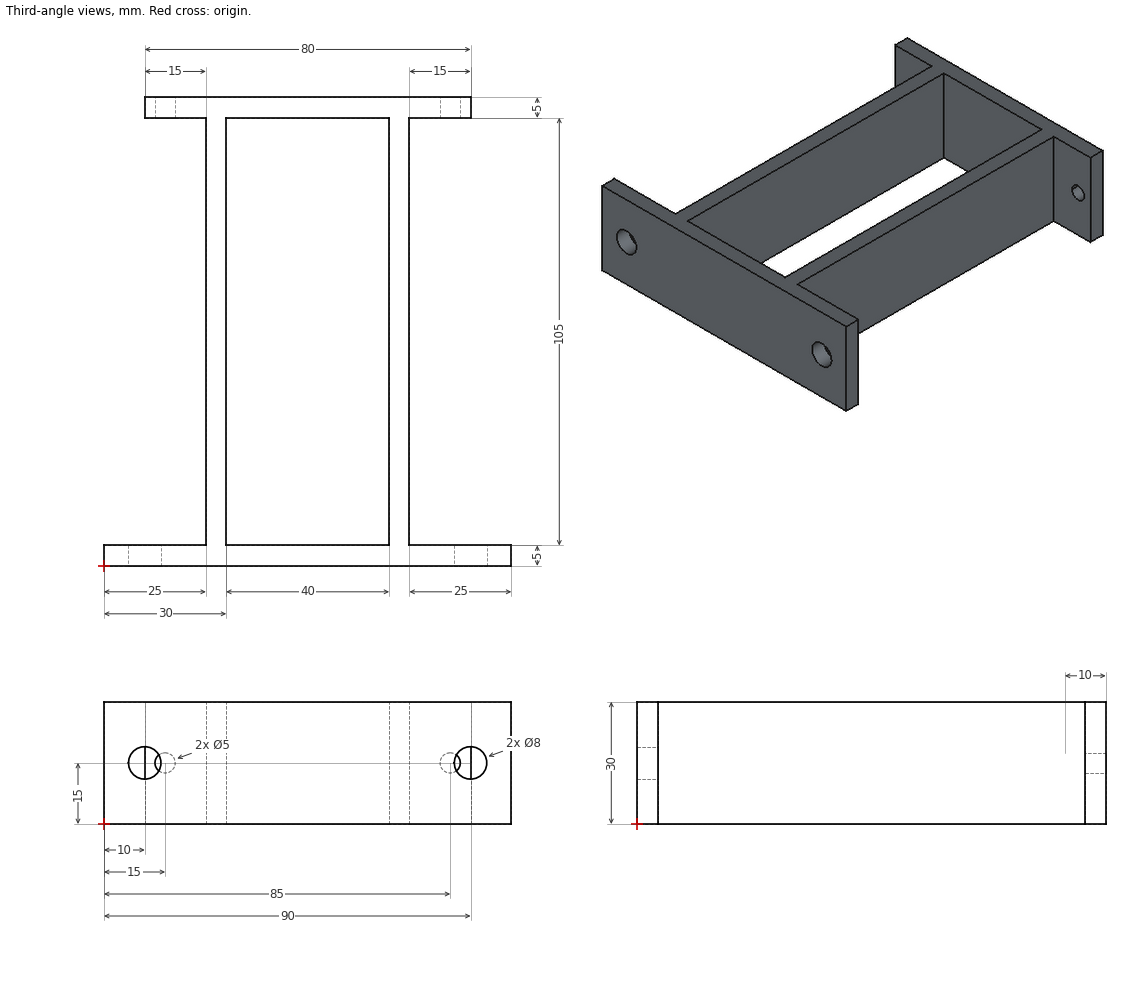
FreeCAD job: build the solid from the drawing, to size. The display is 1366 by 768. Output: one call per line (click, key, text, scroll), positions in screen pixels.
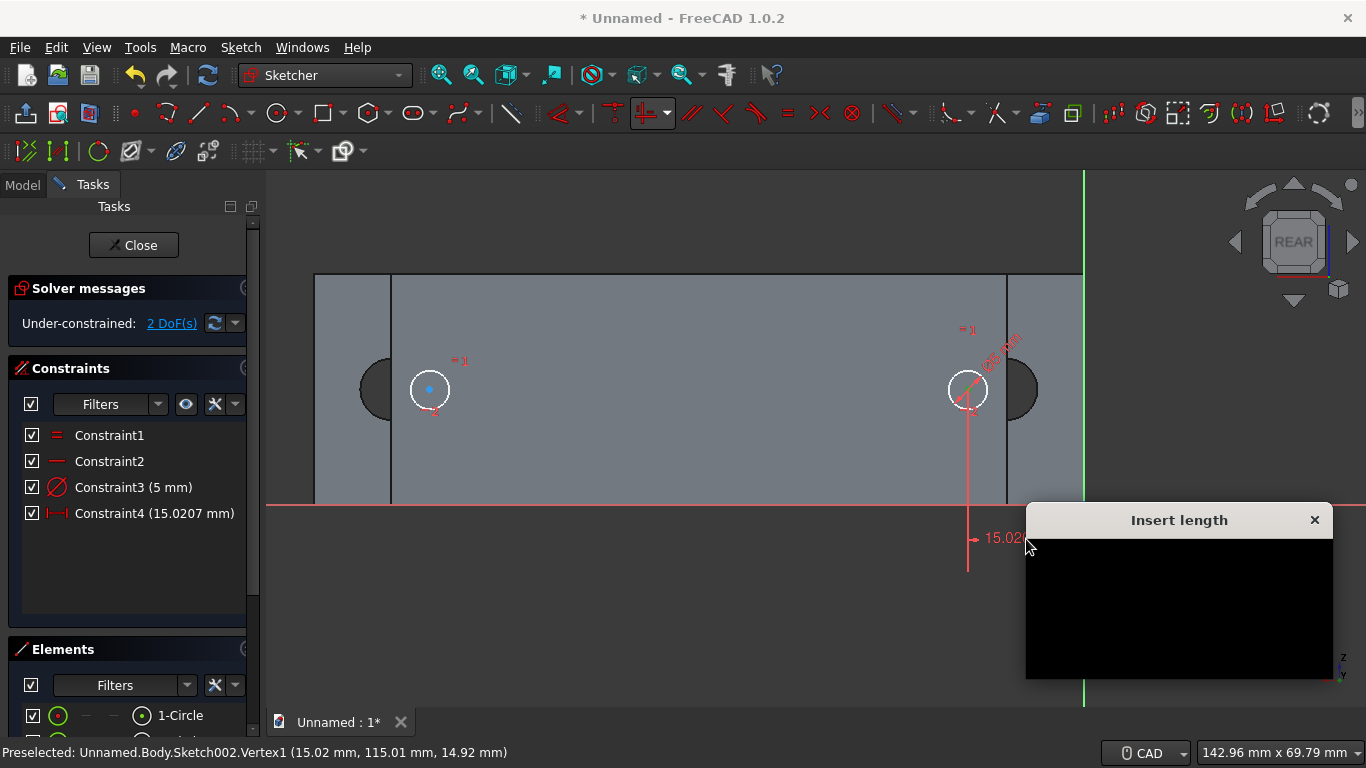
text(15)
key(Return)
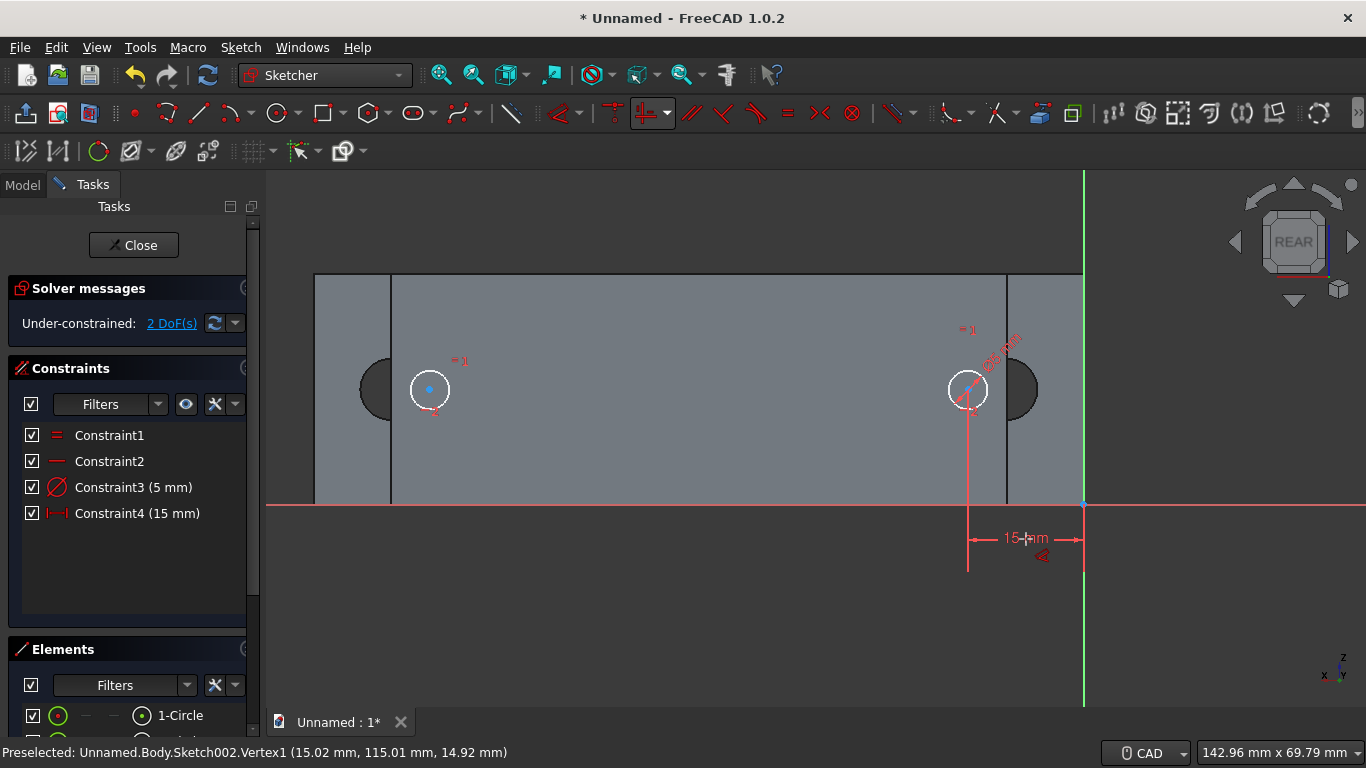
click(968, 390)
click(1118, 447)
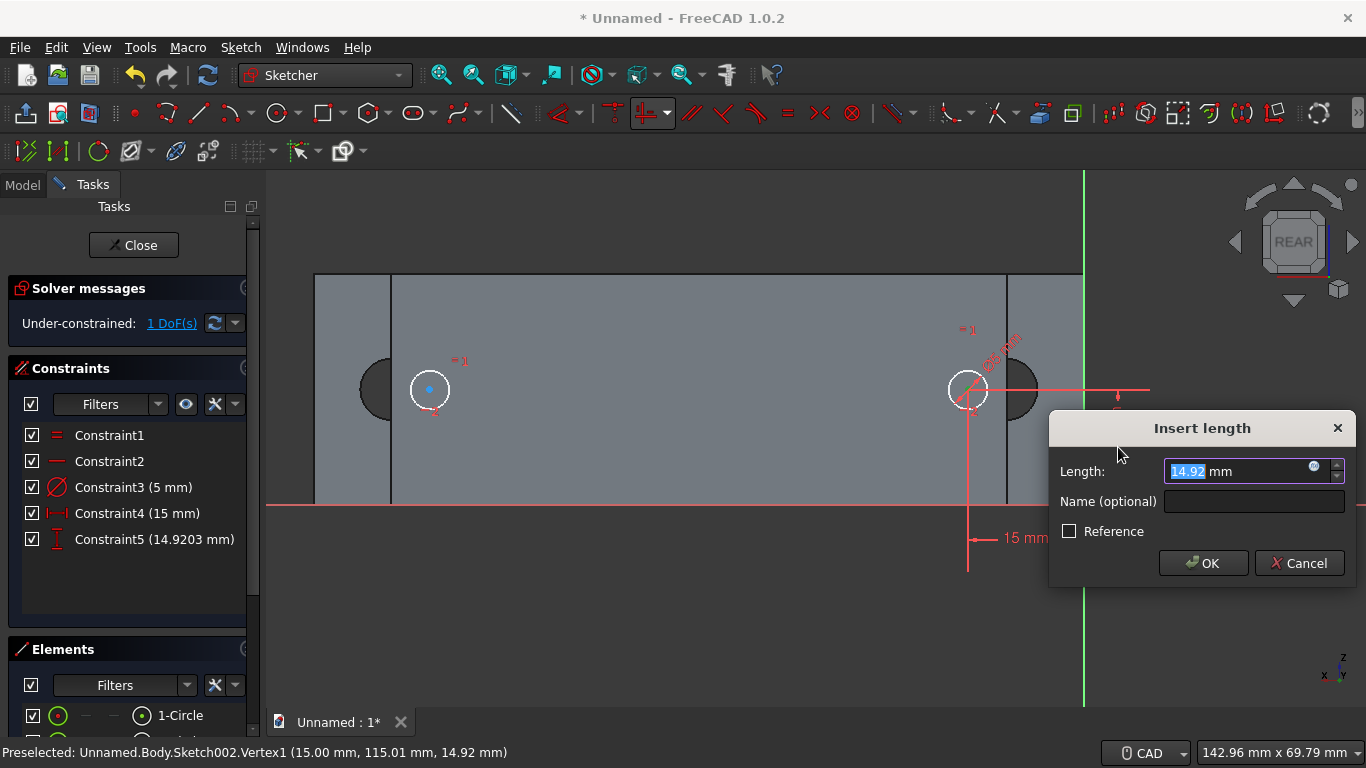
text(15)
key(Return)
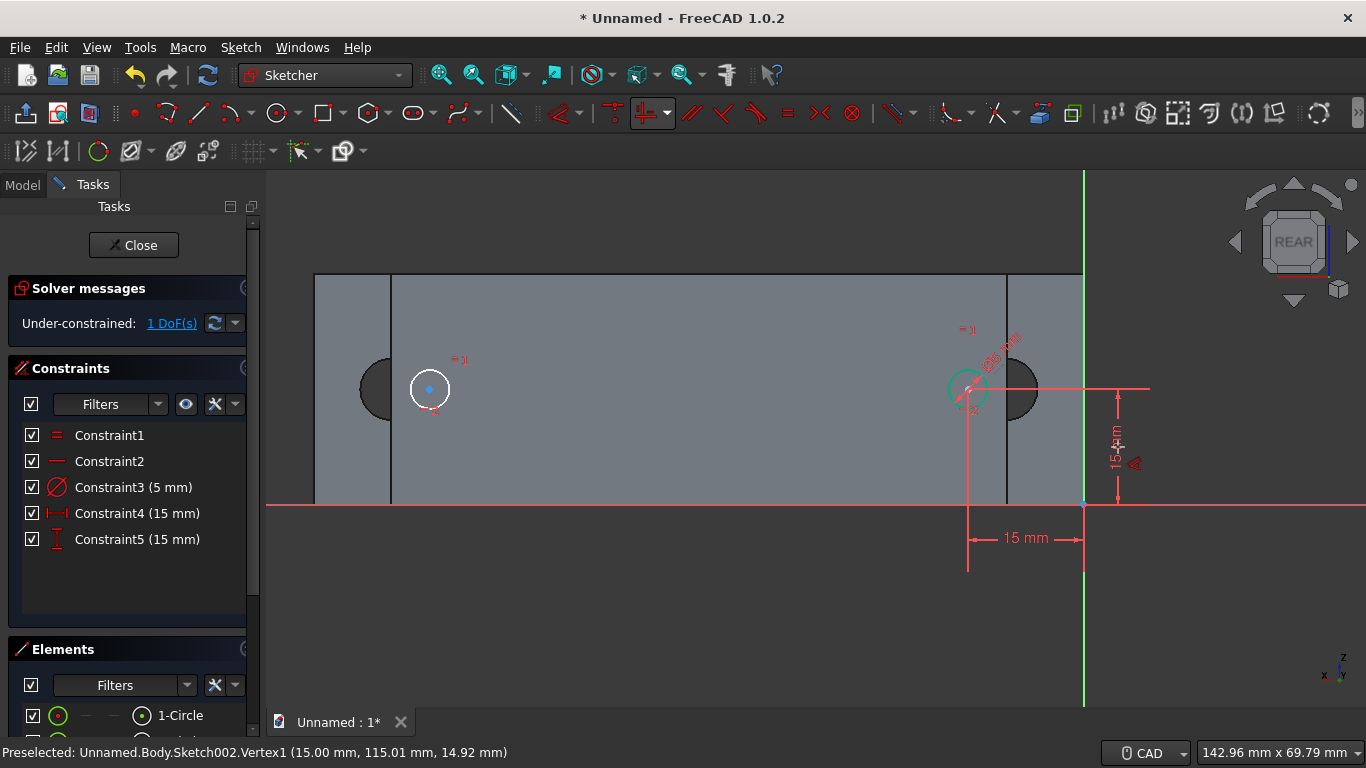
click(430, 389)
click(757, 539)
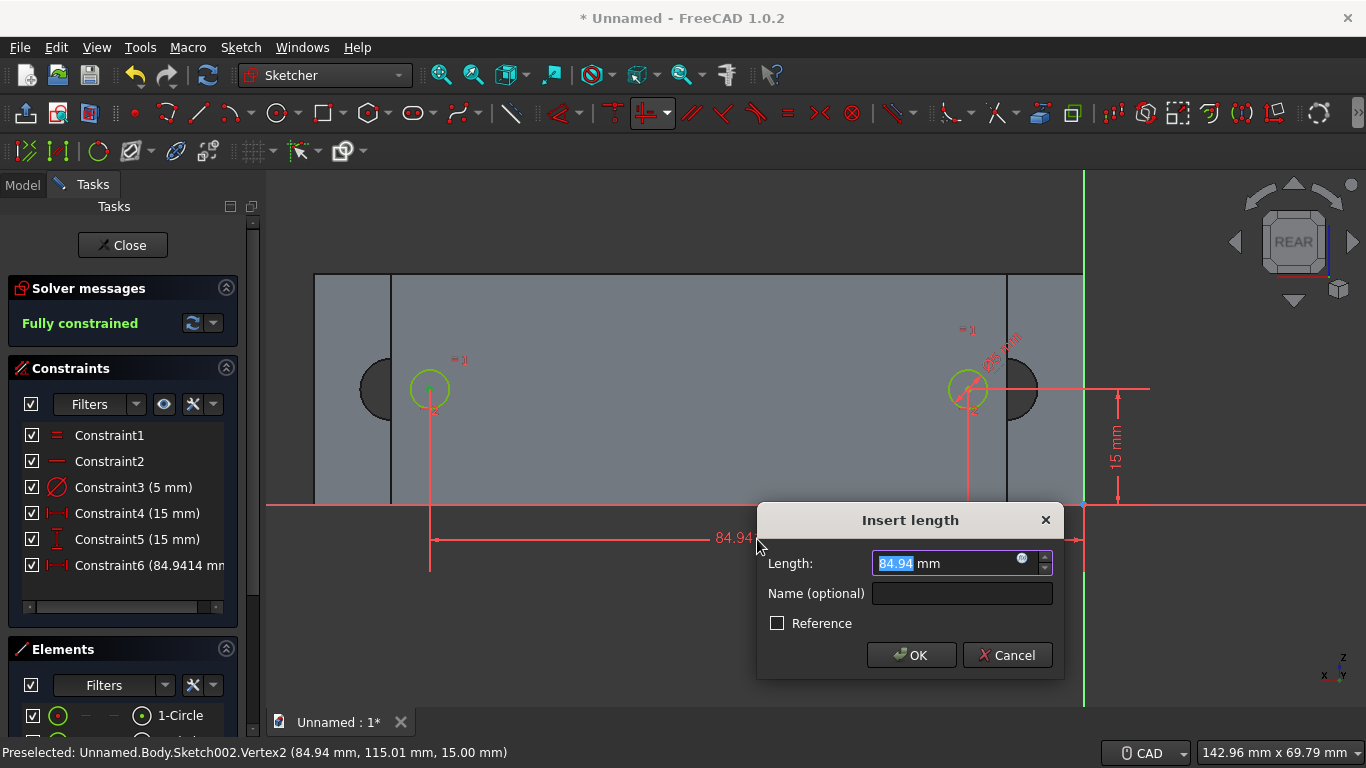
text(85)
key(Return)
key(Escape)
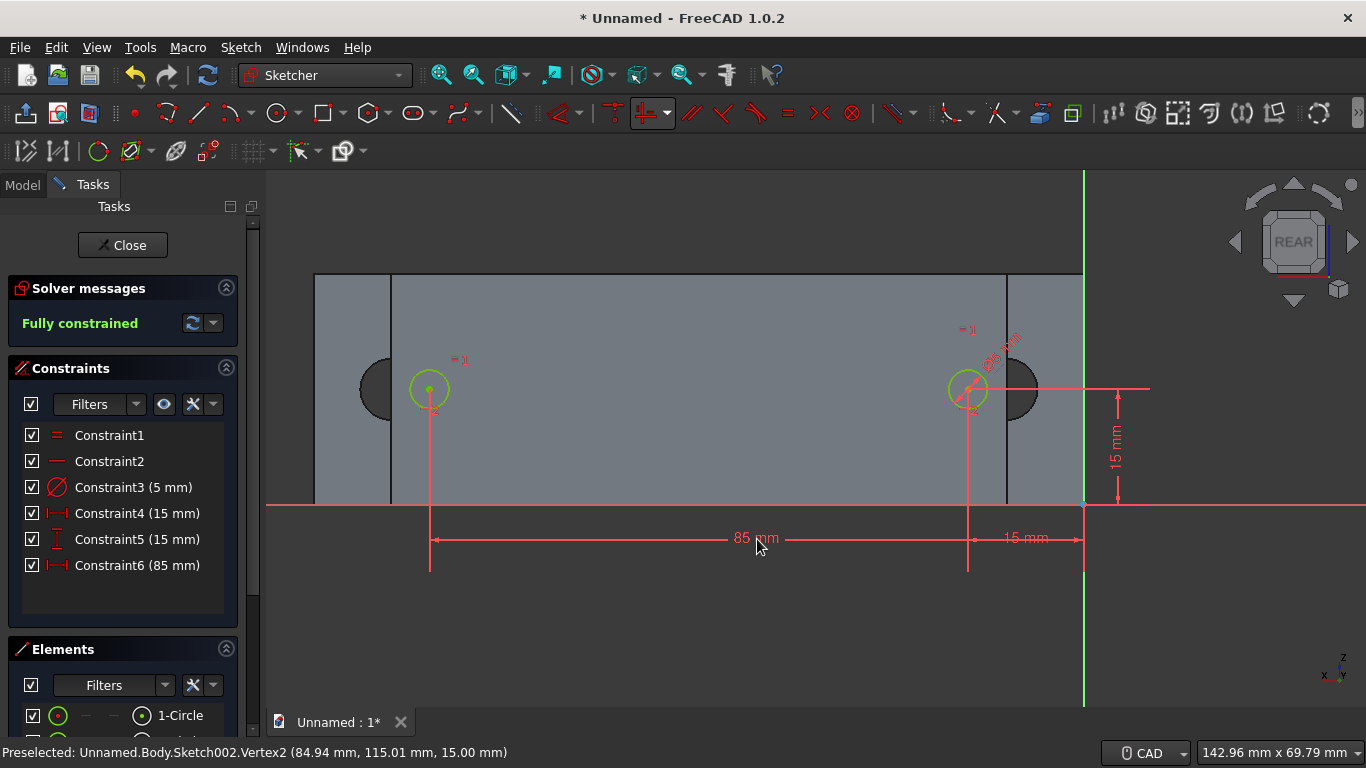
click(123, 245)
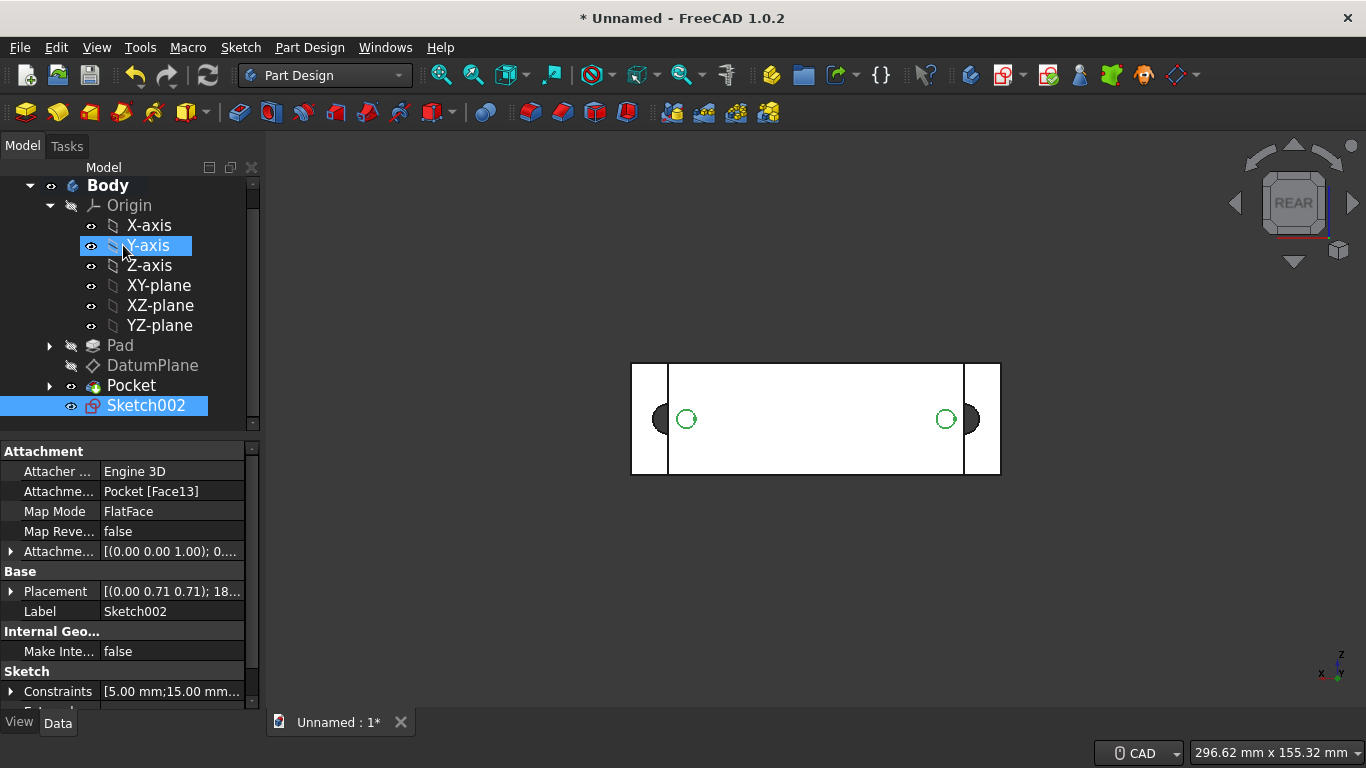
click(240, 112)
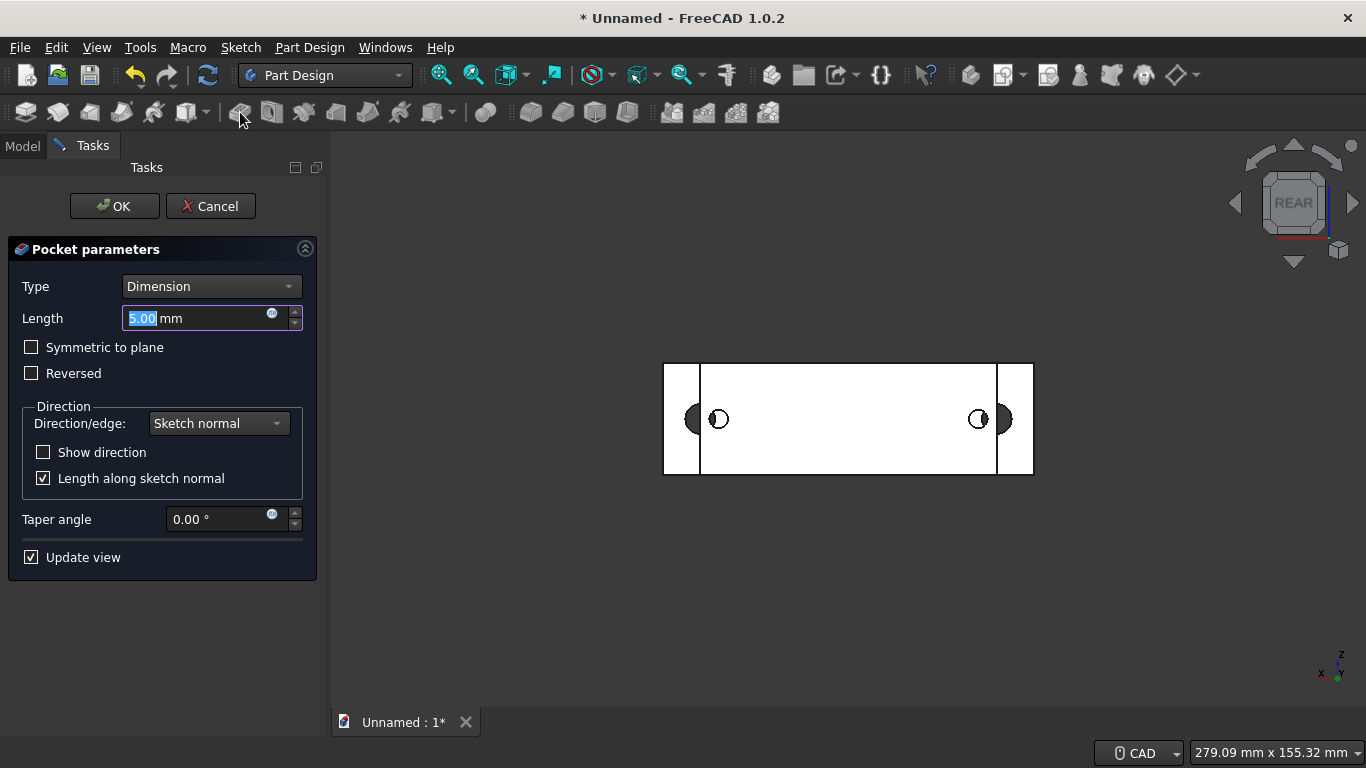
text(10)
key(Tab)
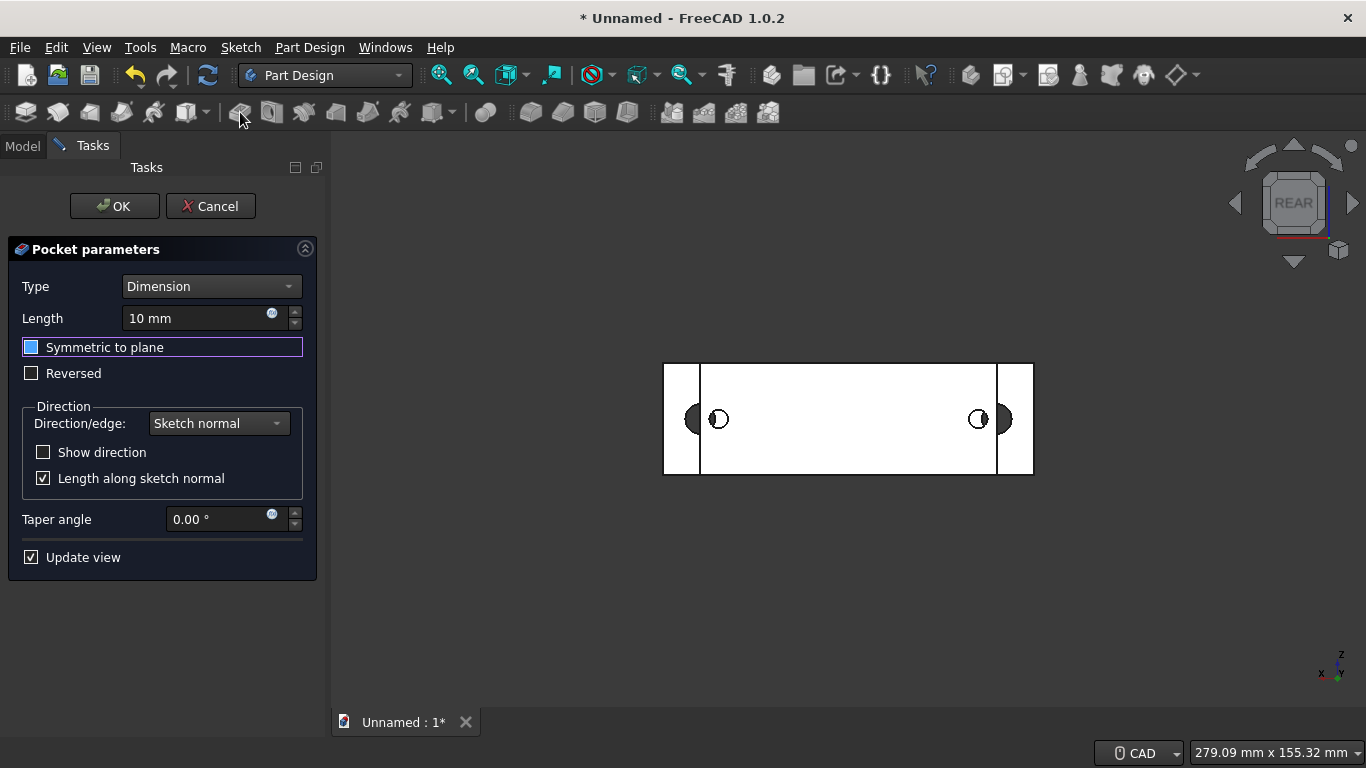
click(115, 206)